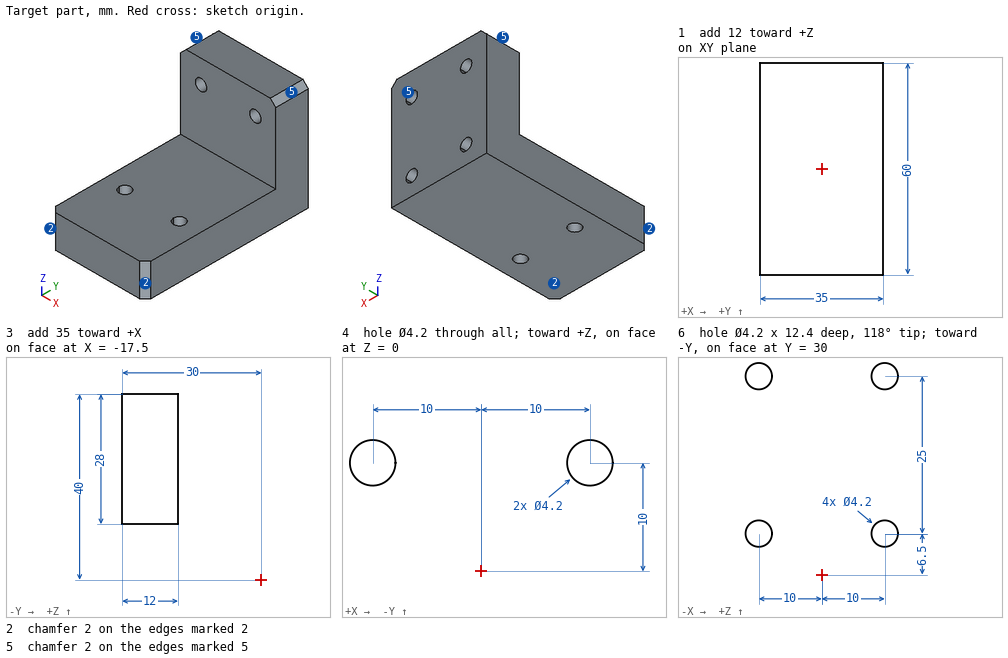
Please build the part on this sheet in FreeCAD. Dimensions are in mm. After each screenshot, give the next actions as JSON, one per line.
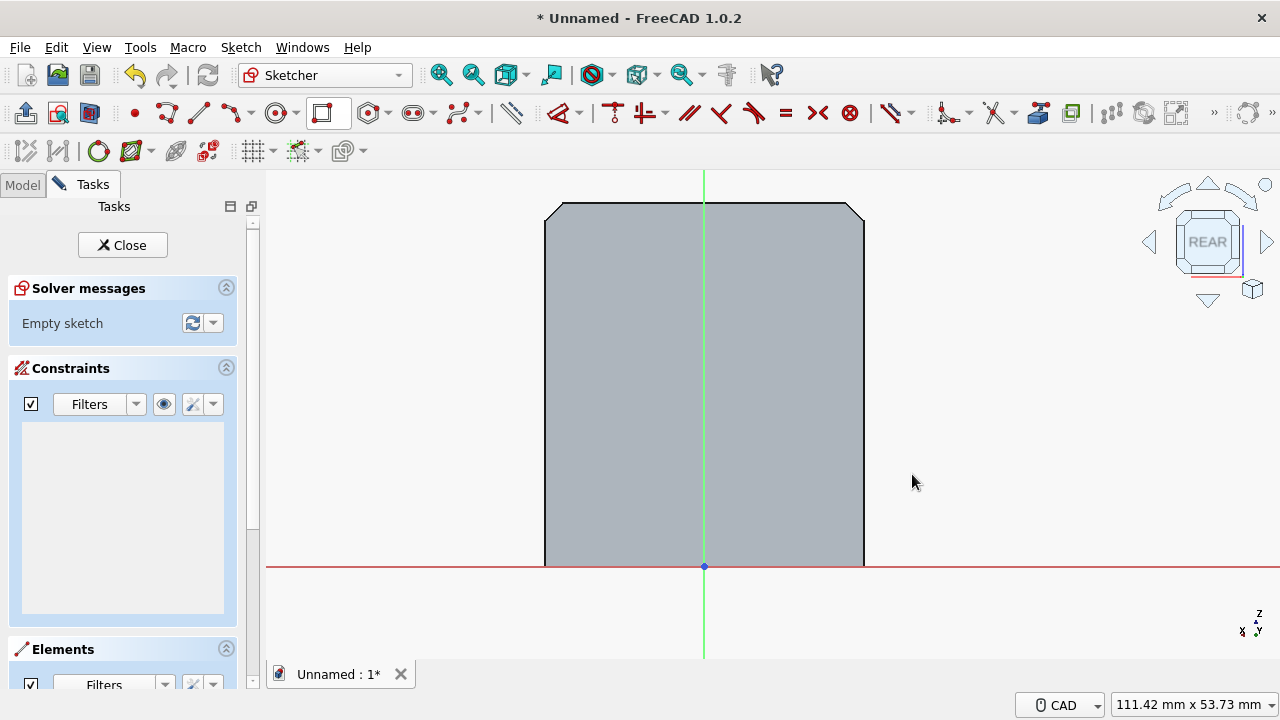
{"action": "left_click", "coordinate": [276, 114]}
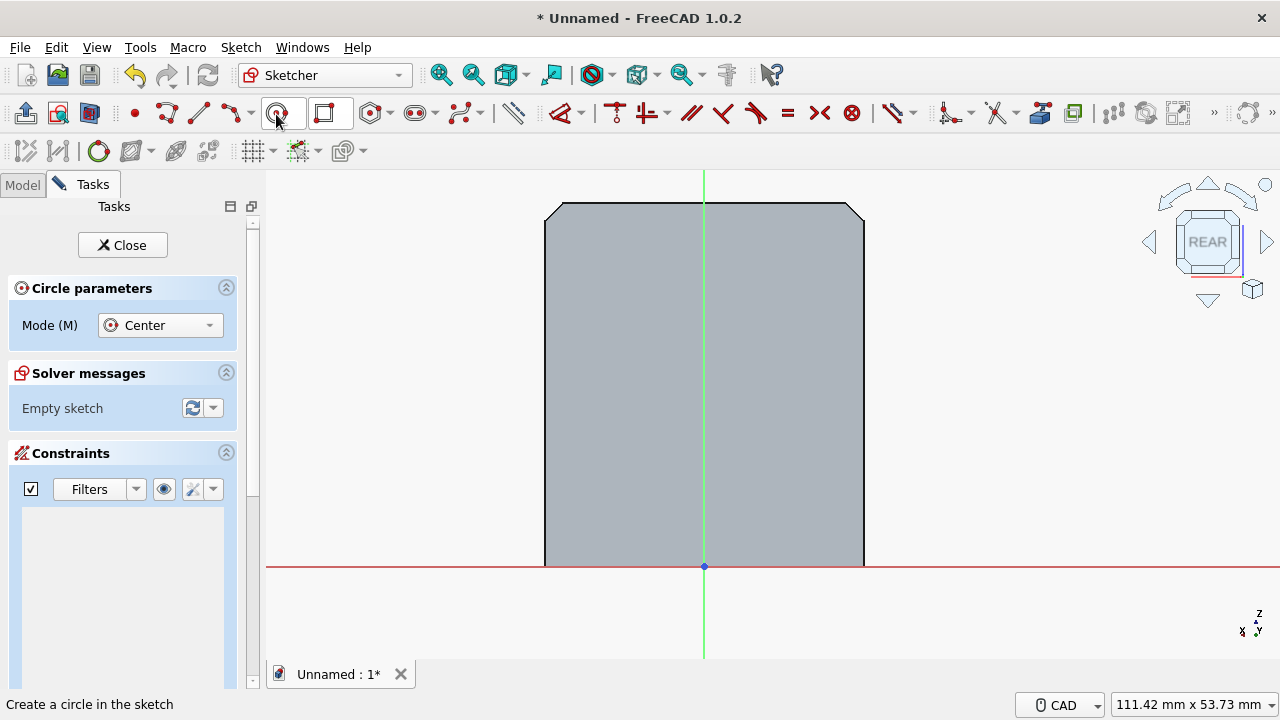
{"action": "left_click", "coordinate": [795, 508]}
{"action": "left_click", "coordinate": [809, 494]}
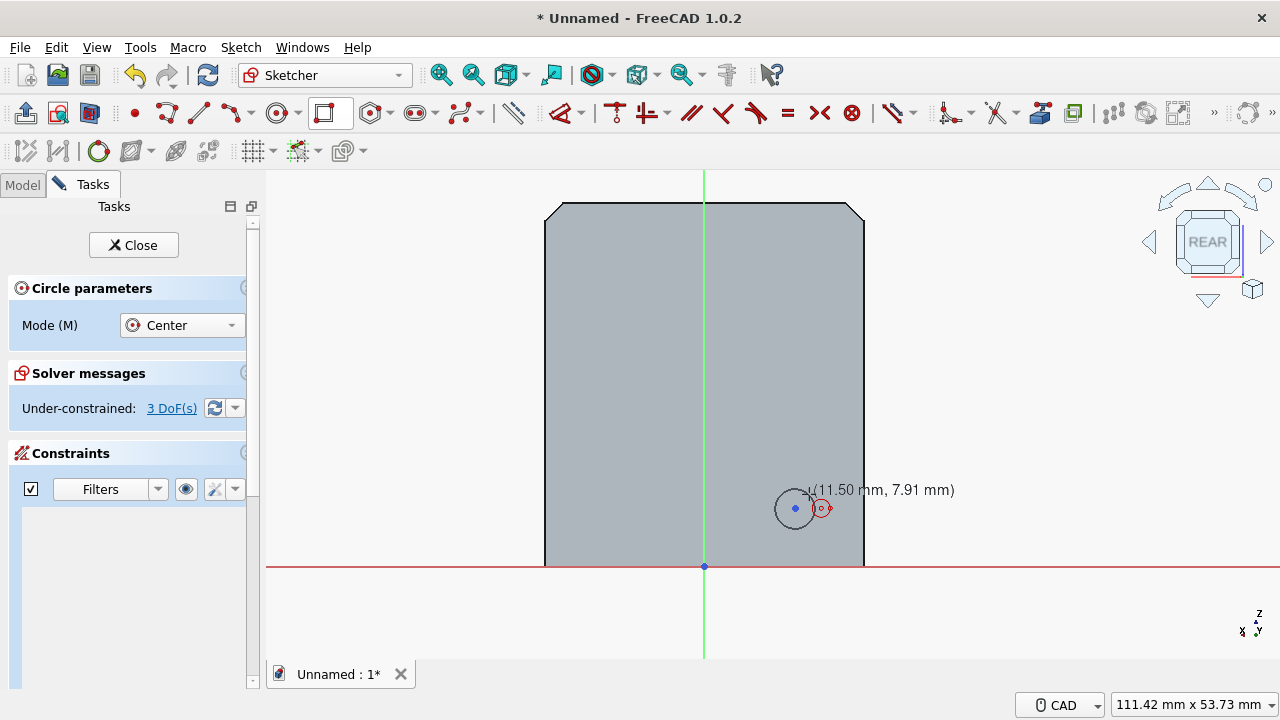
{"action": "left_click", "coordinate": [613, 508]}
{"action": "left_click", "coordinate": [627, 494]}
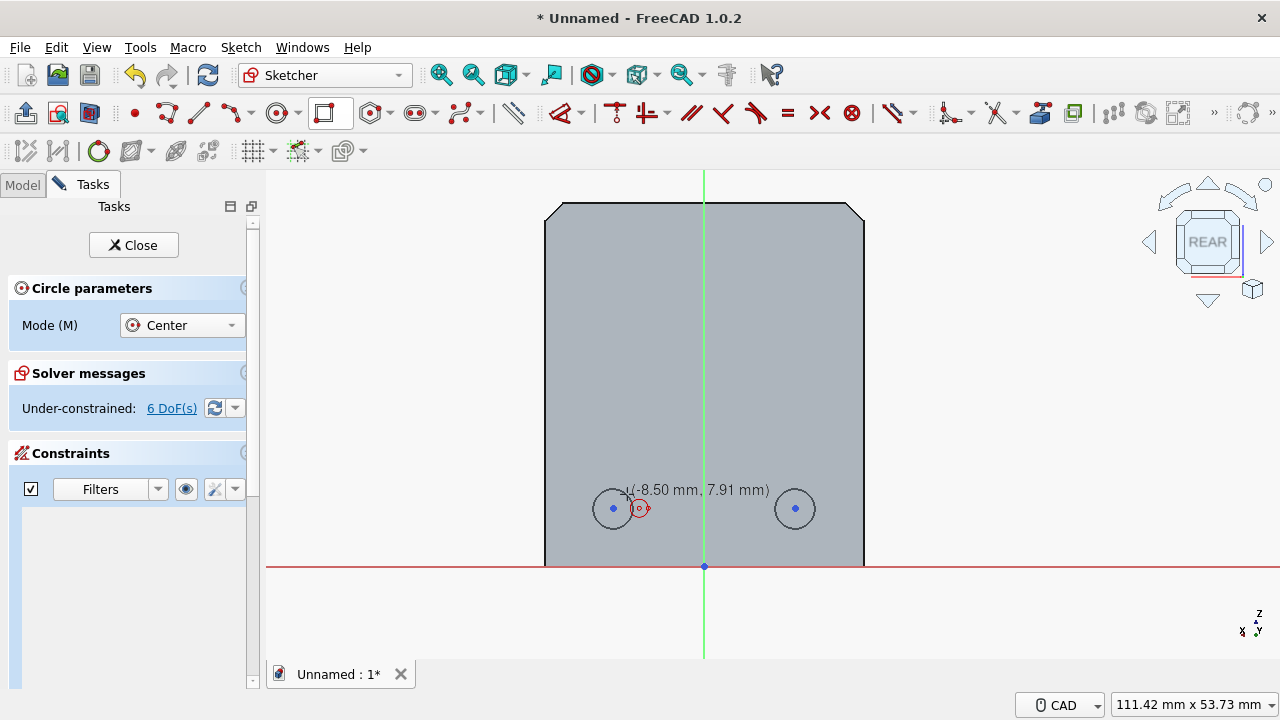
{"action": "left_click", "coordinate": [795, 280]}
{"action": "left_click", "coordinate": [809, 267]}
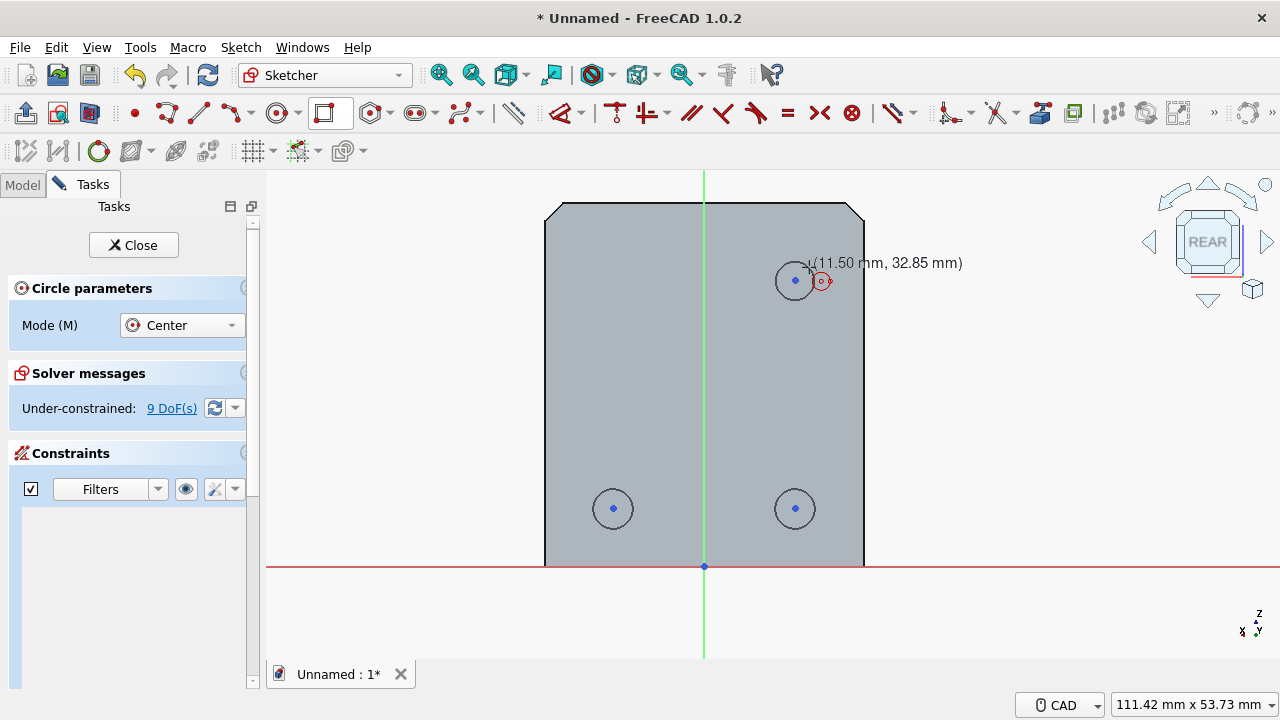
{"action": "left_click", "coordinate": [613, 280]}
{"action": "left_click", "coordinate": [627, 267]}
{"action": "key", "text": "Escape"}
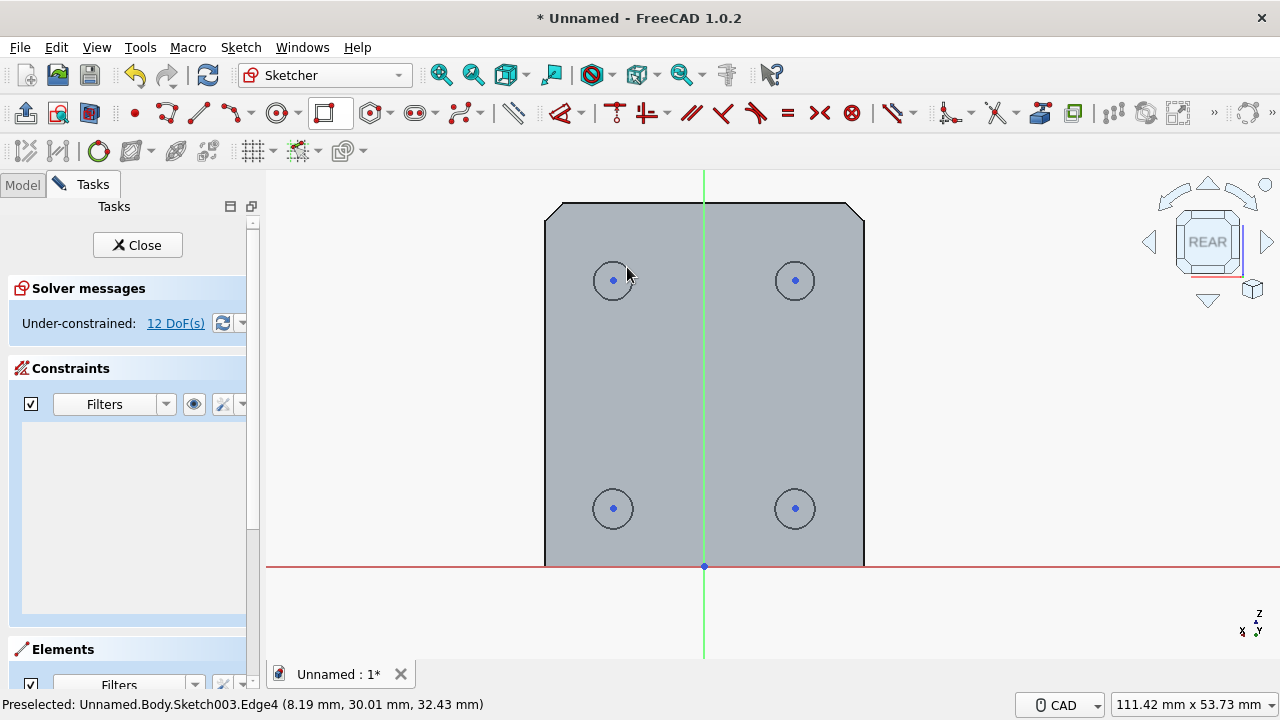
{"action": "left_click", "coordinate": [809, 495]}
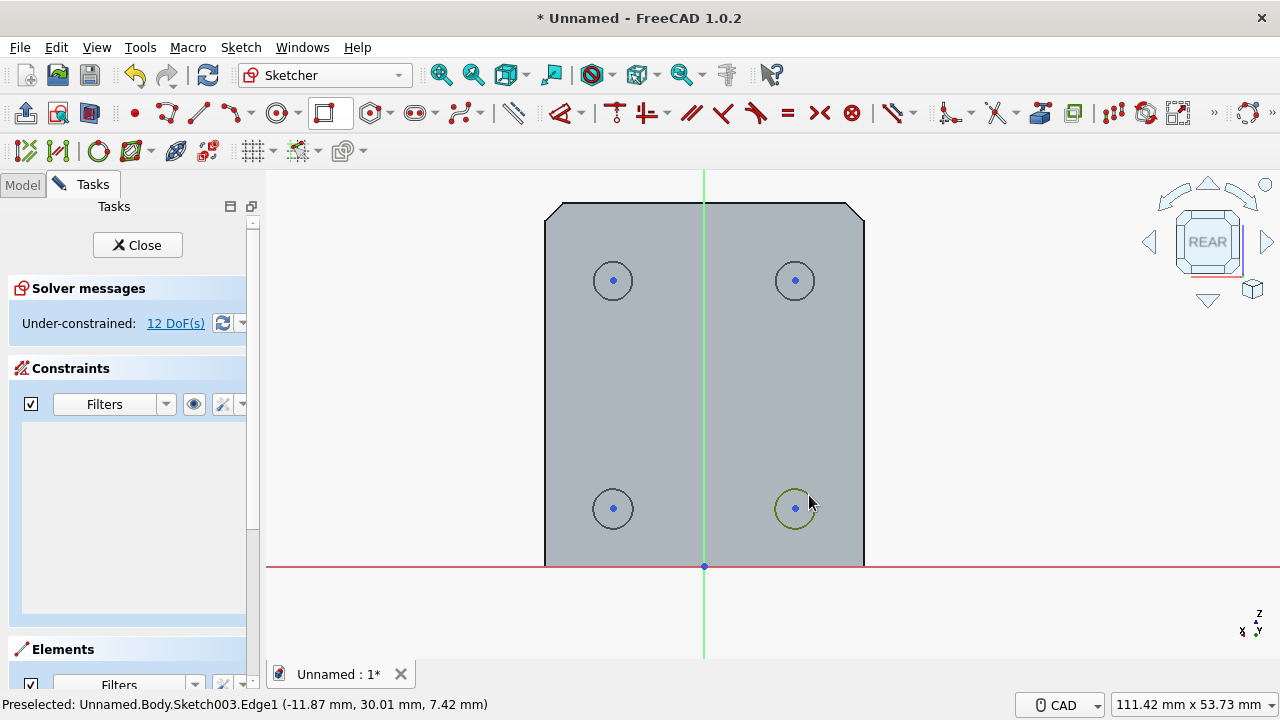
{"action": "left_click", "coordinate": [627, 495]}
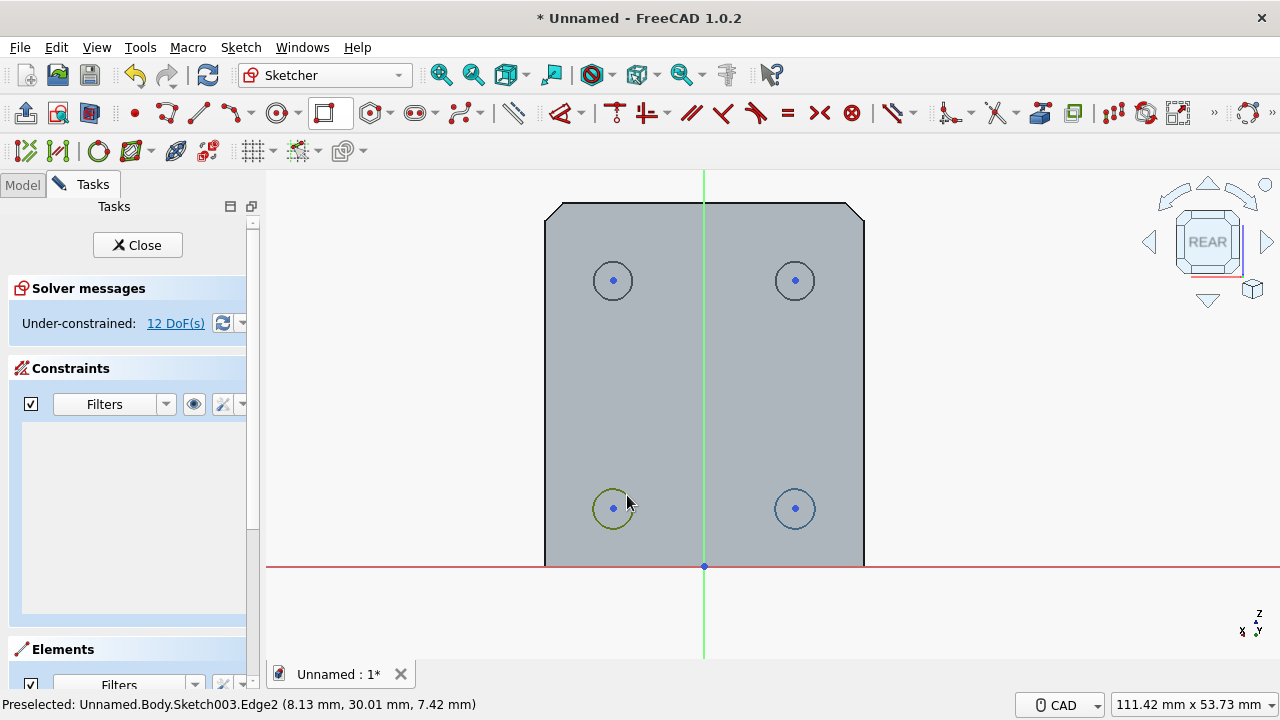
{"action": "left_click", "coordinate": [808, 267]}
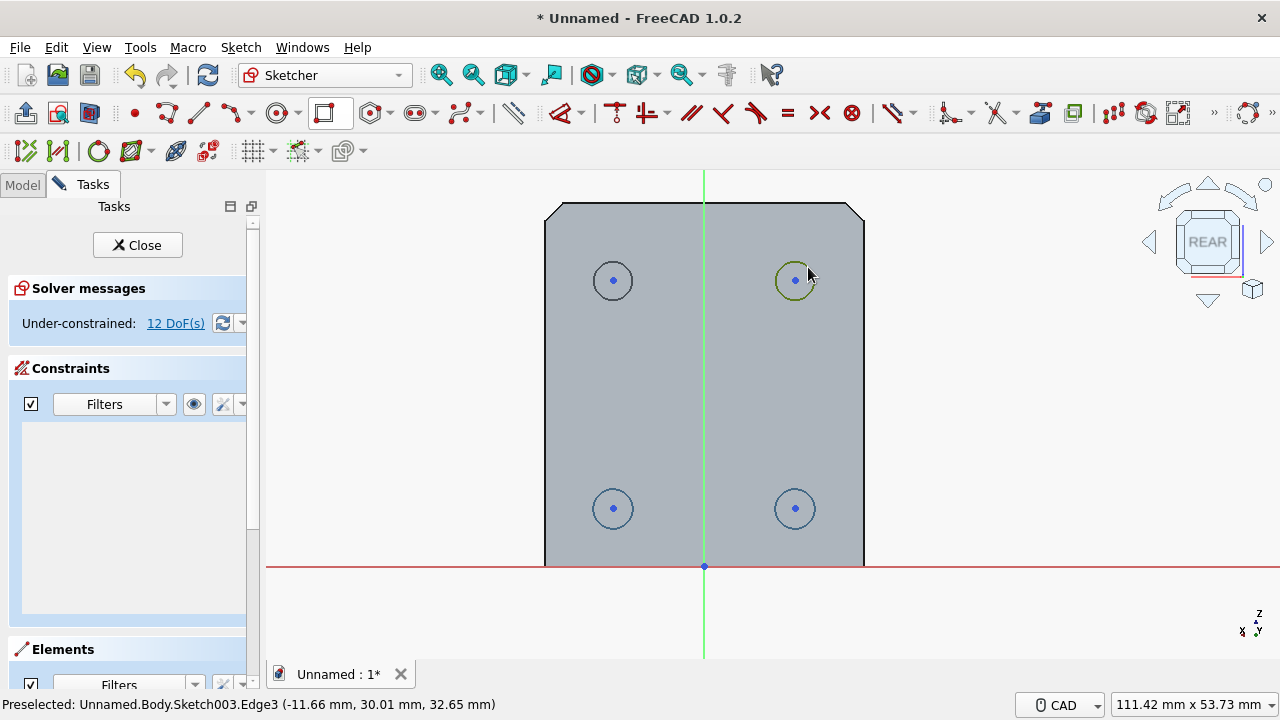
{"action": "left_click", "coordinate": [626, 267]}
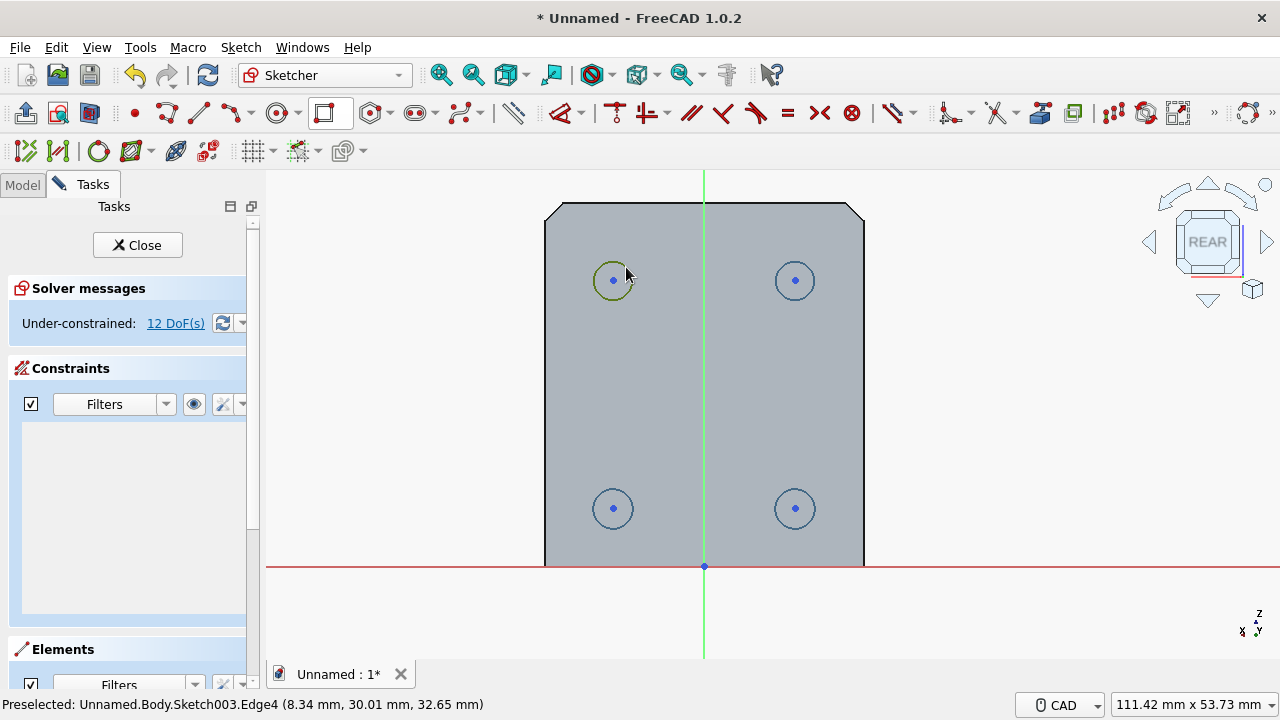
{"action": "left_click", "coordinate": [788, 114]}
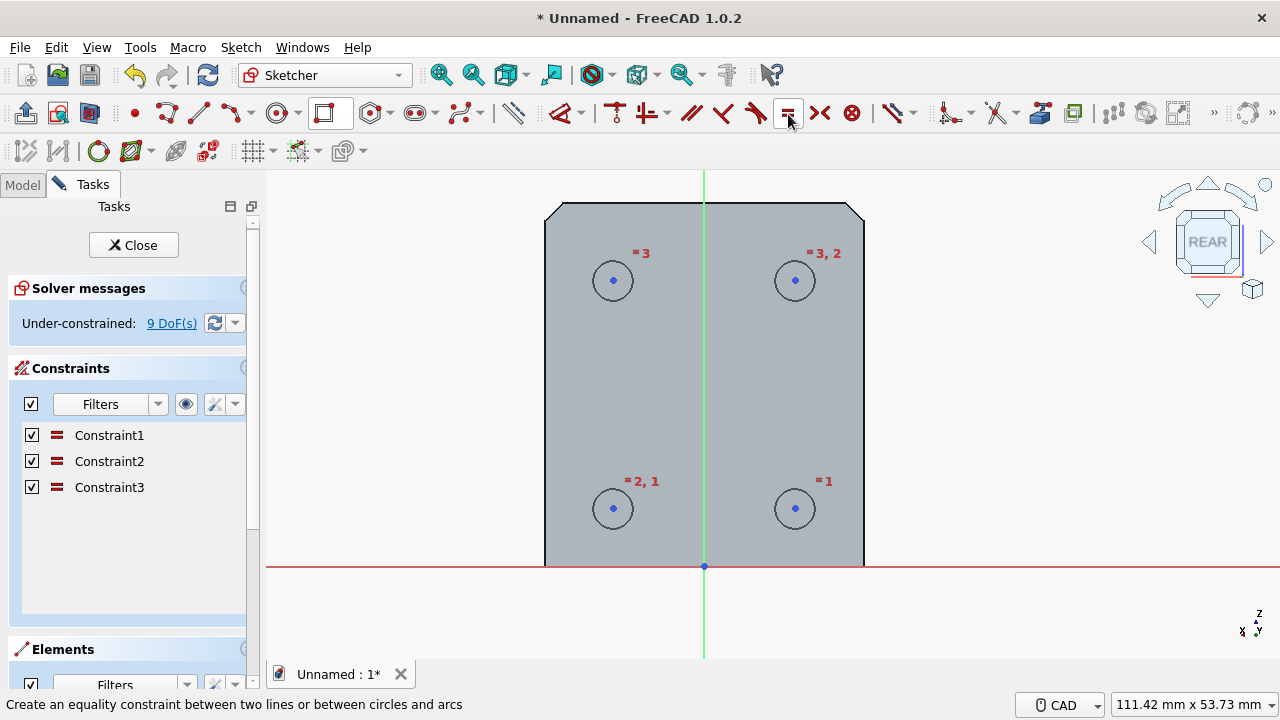
{"action": "left_click", "coordinate": [795, 509]}